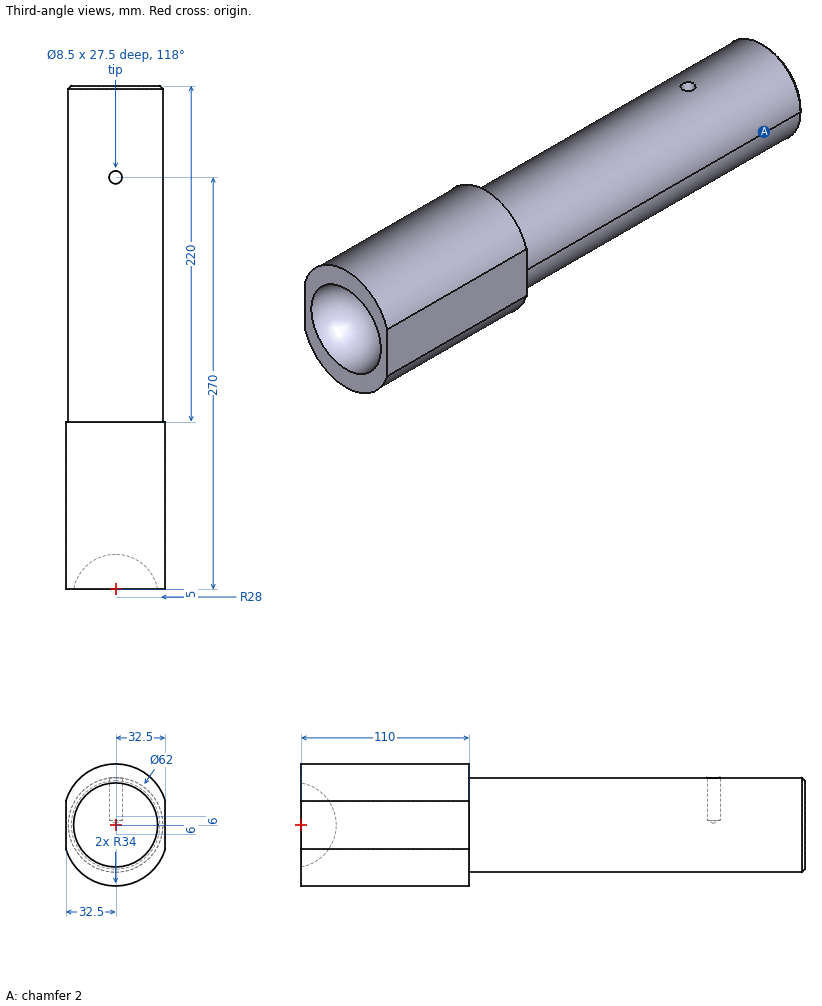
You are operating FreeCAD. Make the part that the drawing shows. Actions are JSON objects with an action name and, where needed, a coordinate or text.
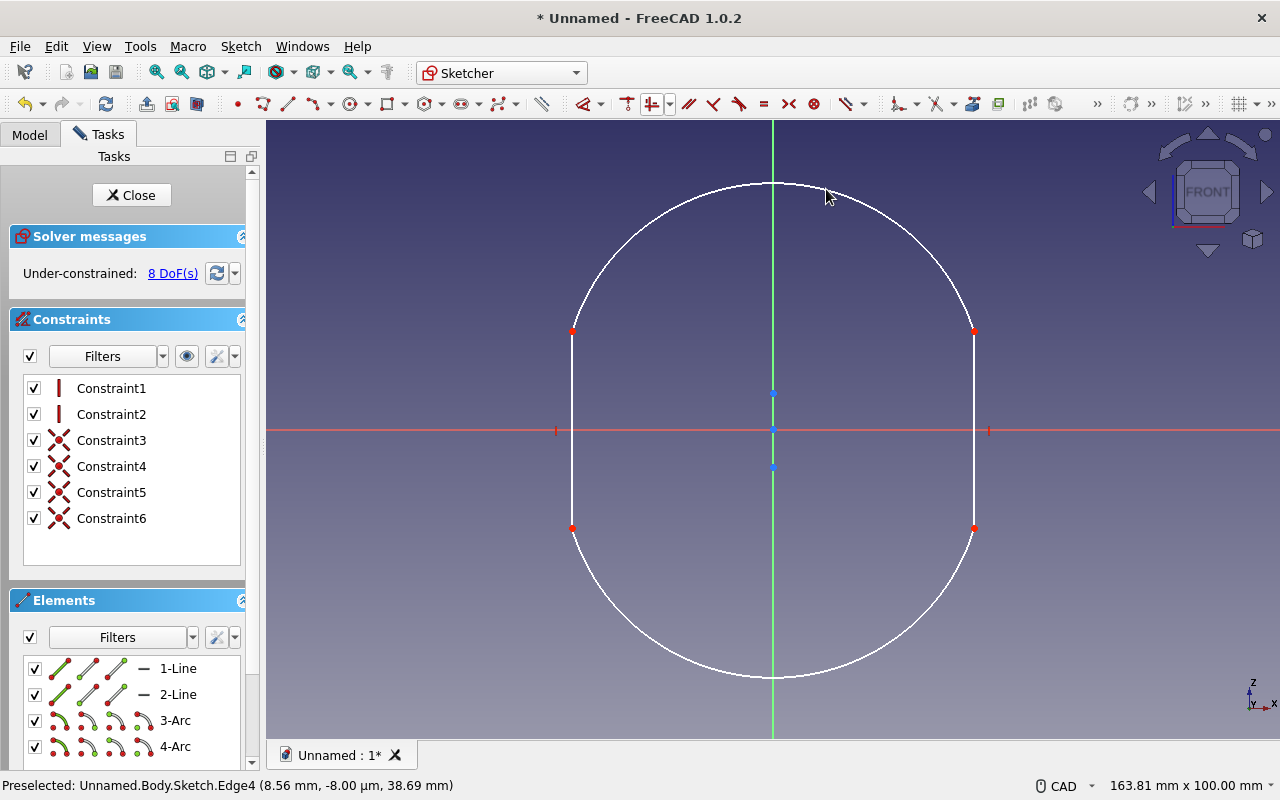
{"action": "left_click", "coordinate": [670, 651]}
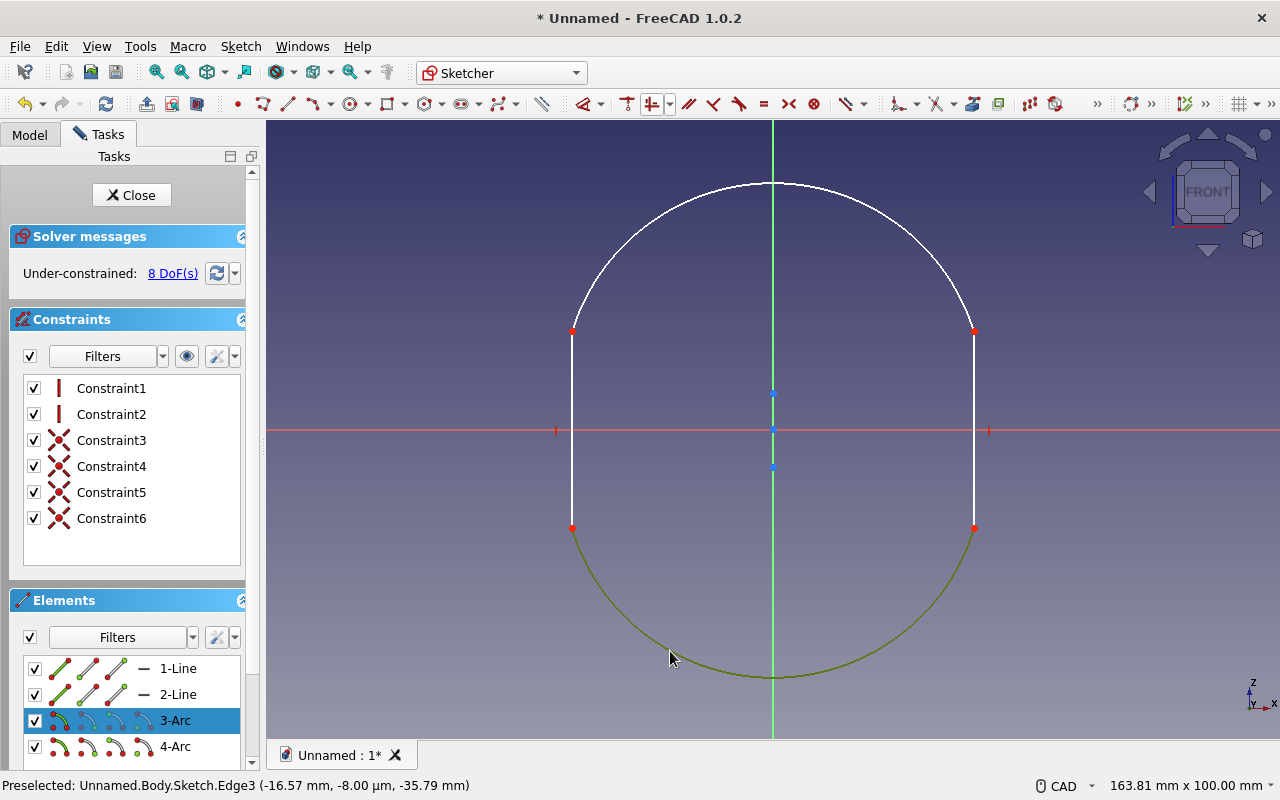
{"action": "left_click", "coordinate": [876, 210]}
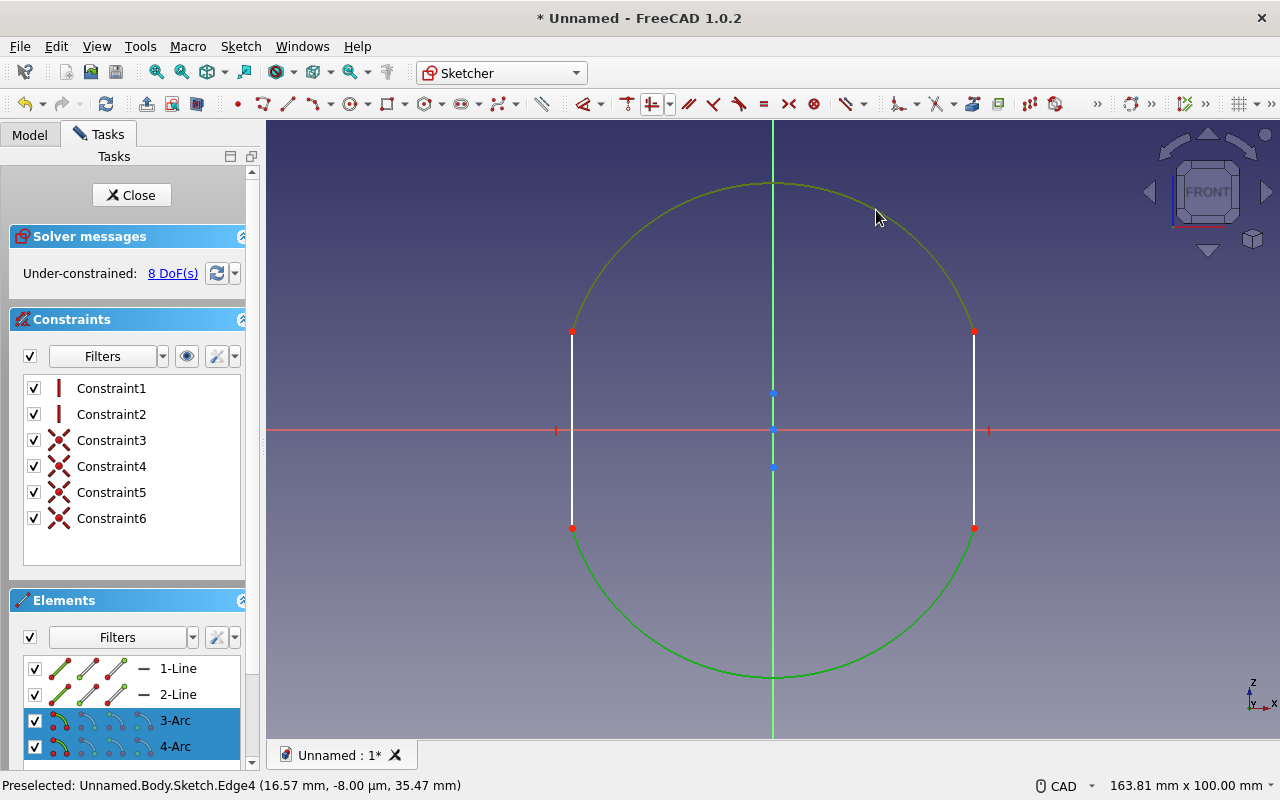
{"action": "left_click", "coordinate": [764, 104]}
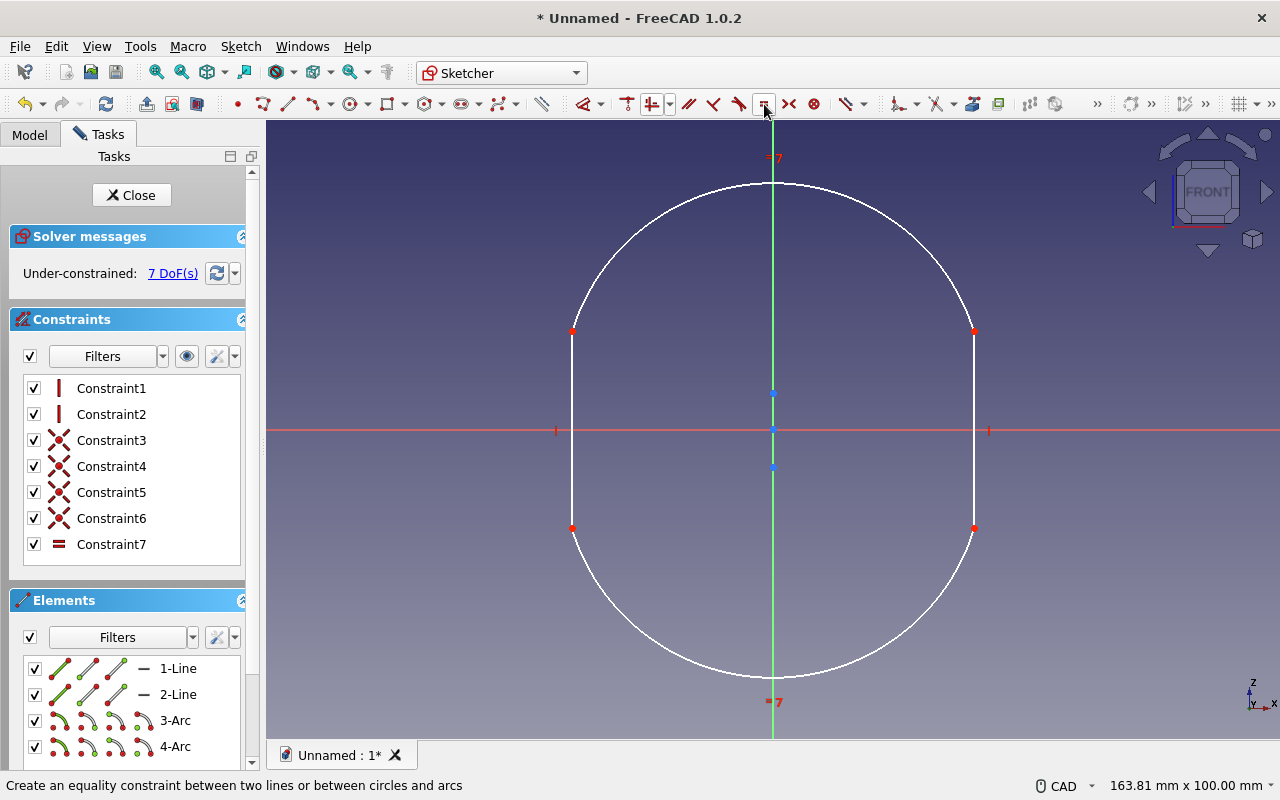
{"action": "left_click", "coordinate": [773, 468]}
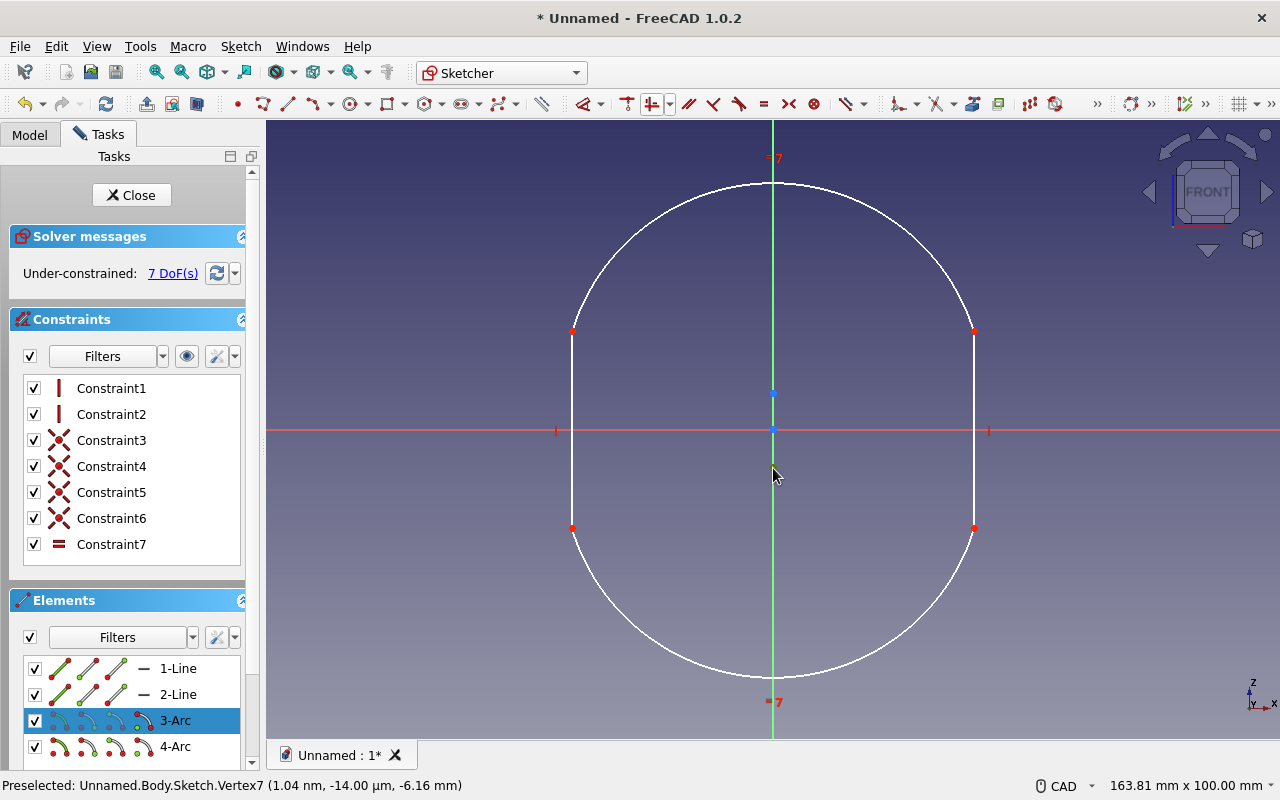
{"action": "left_click", "coordinate": [773, 631]}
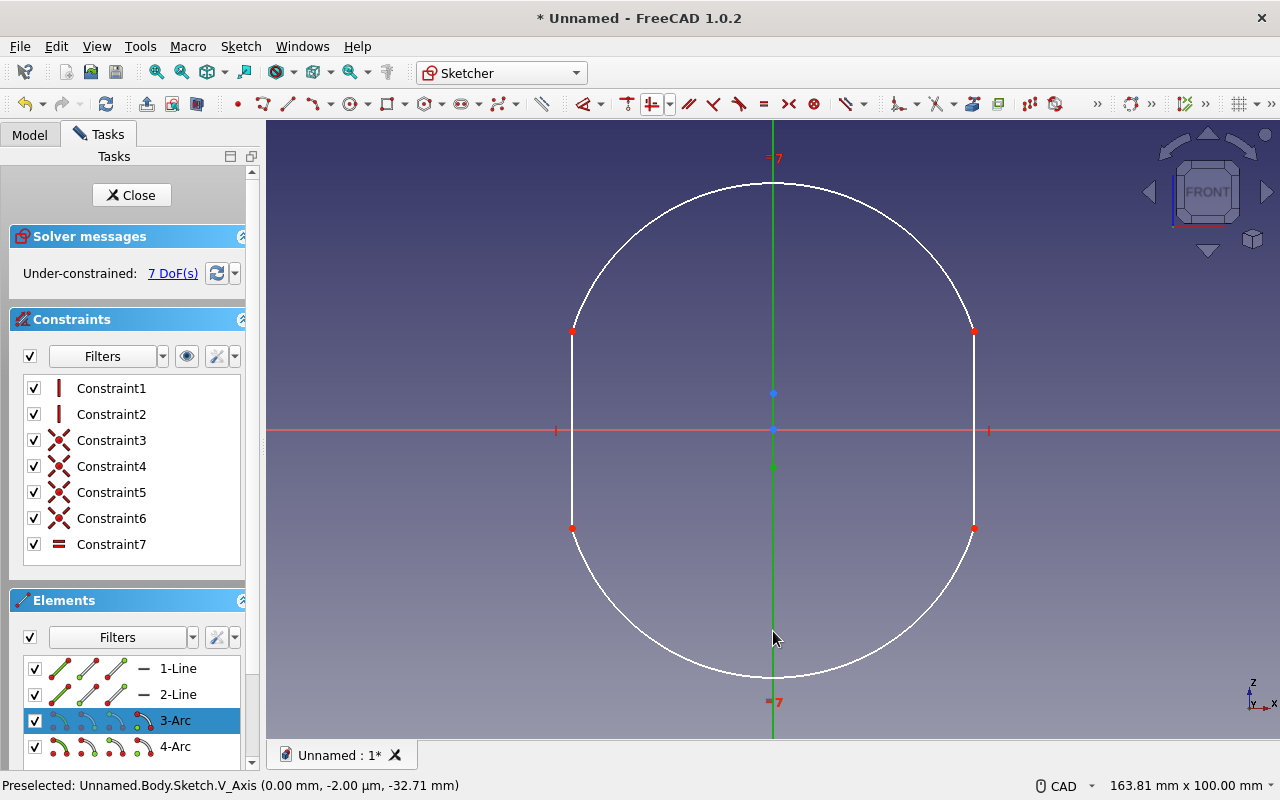
{"action": "left_click", "coordinate": [627, 104]}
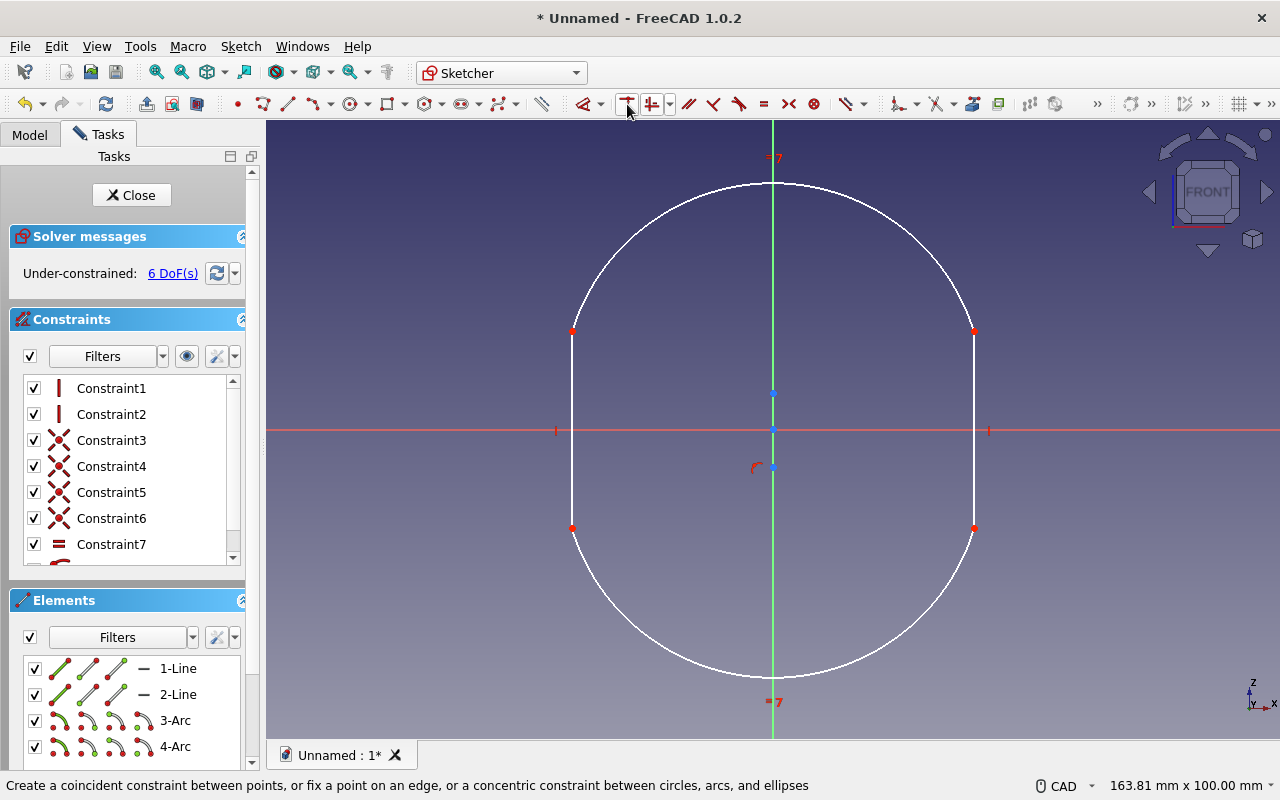
{"action": "left_click", "coordinate": [773, 393]}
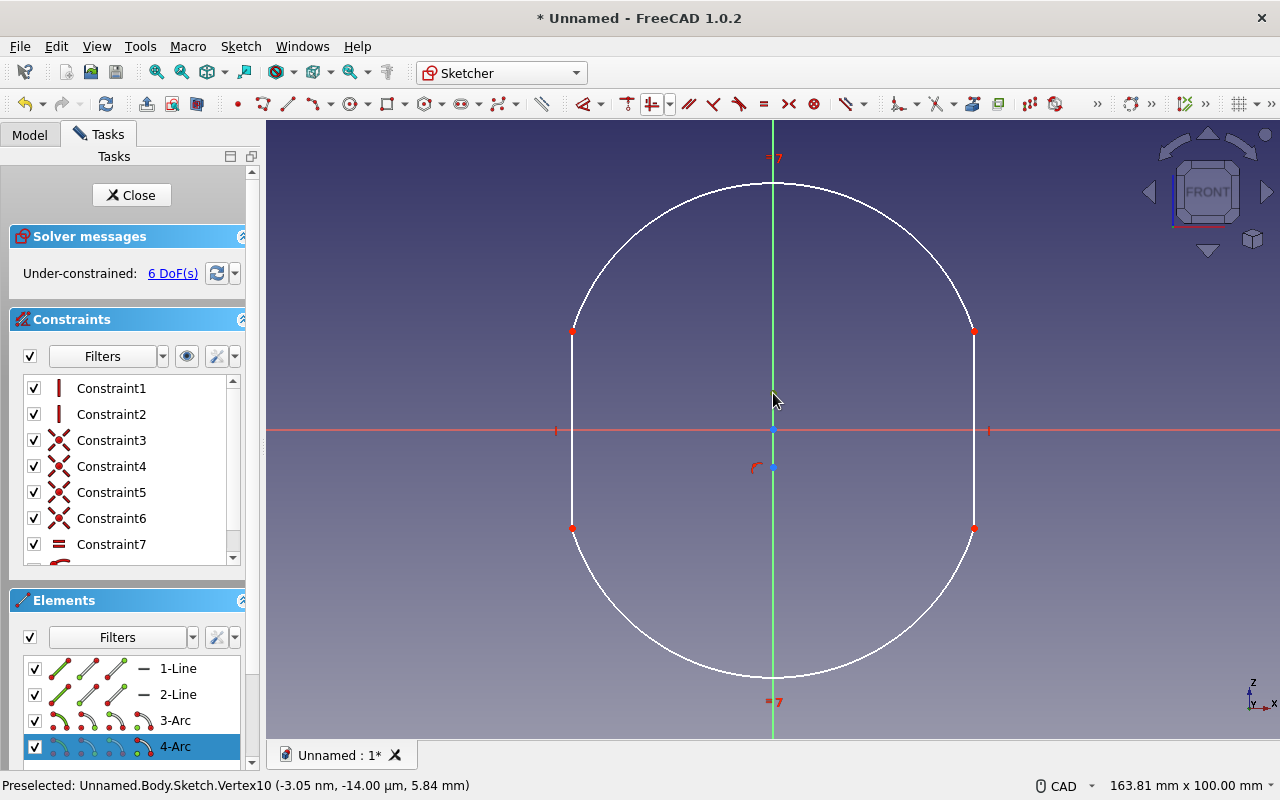
{"action": "left_click", "coordinate": [773, 631]}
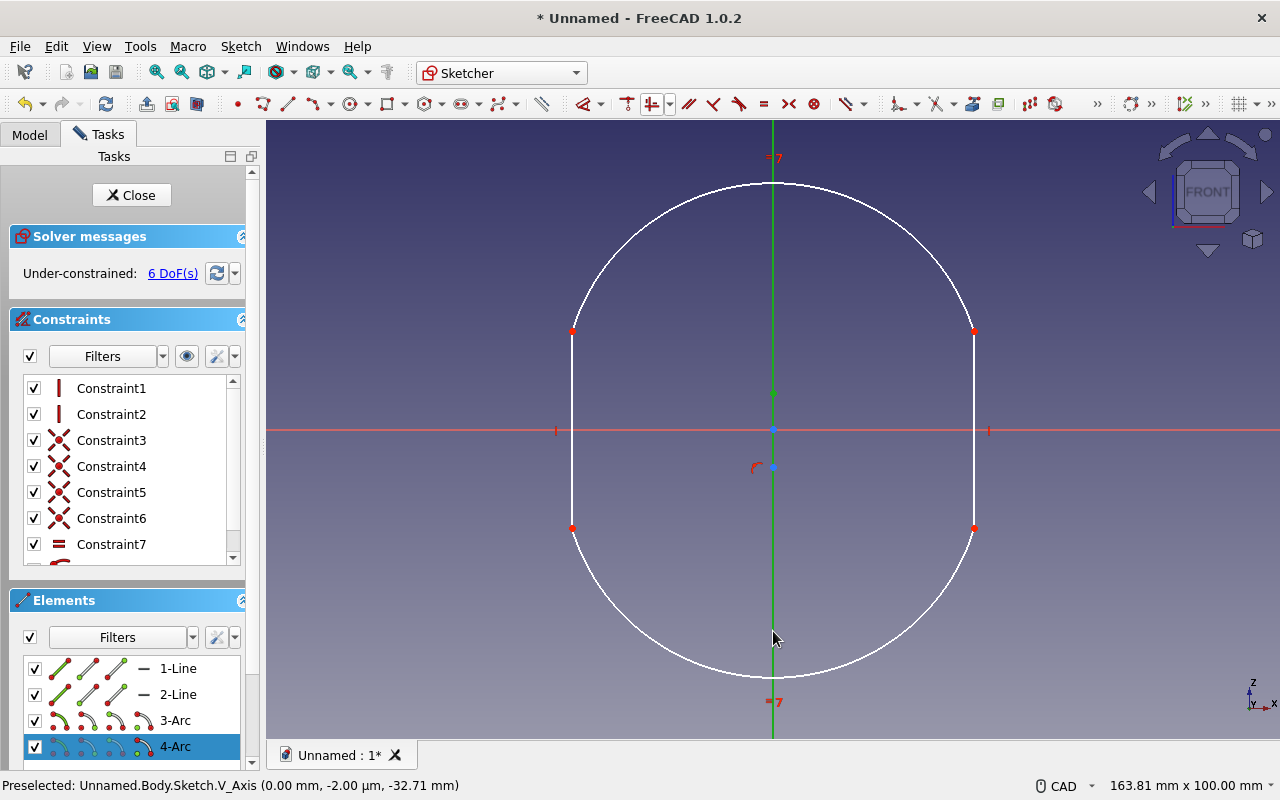
{"action": "left_click", "coordinate": [627, 104]}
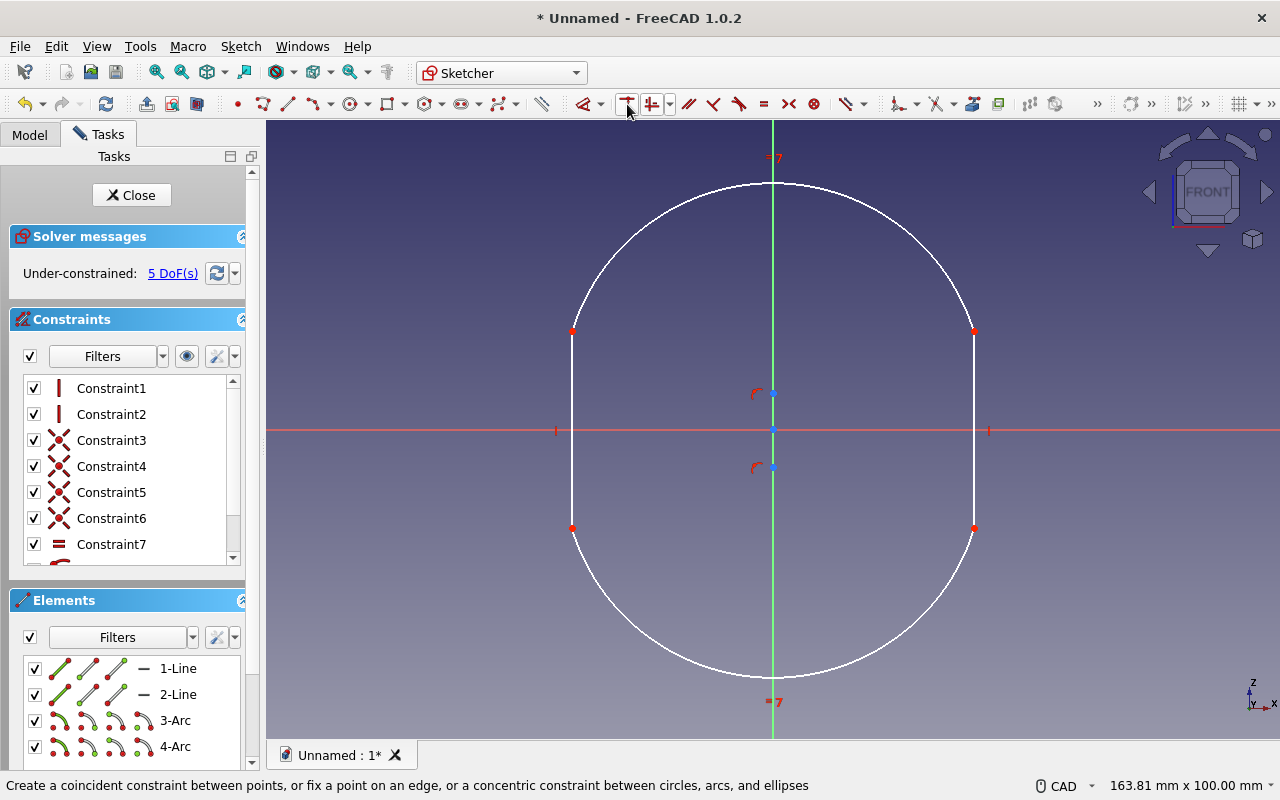
{"action": "key", "text": "d"}